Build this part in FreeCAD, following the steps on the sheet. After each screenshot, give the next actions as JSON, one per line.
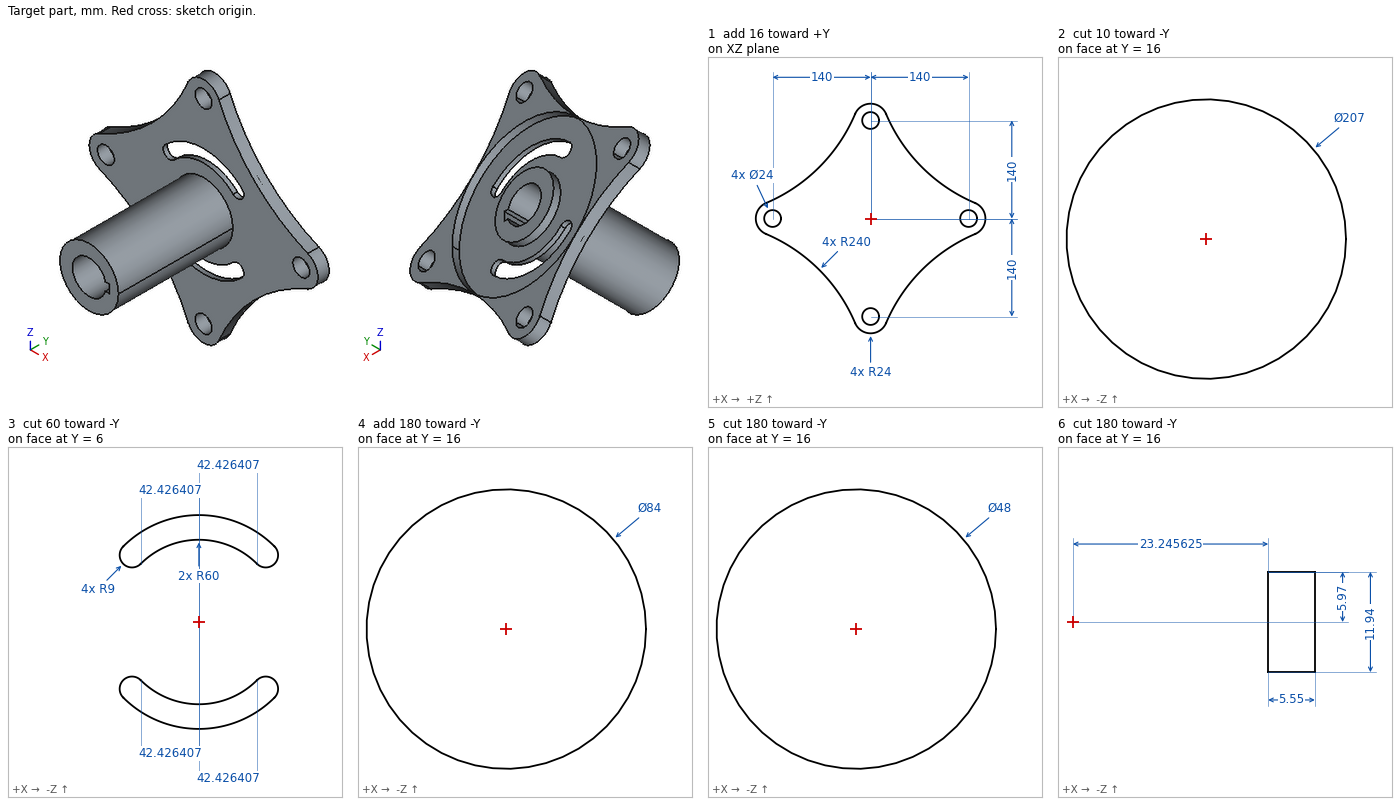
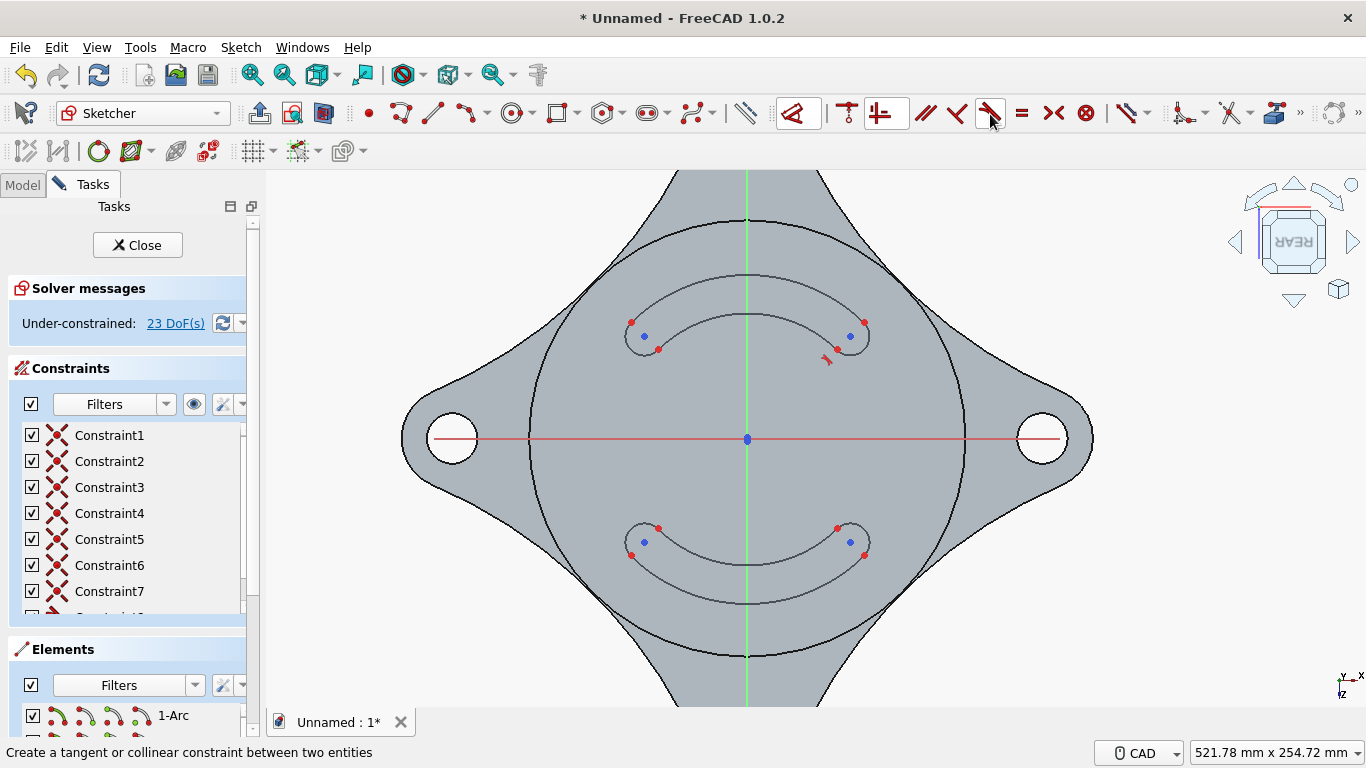
{"action": "left_click", "coordinate": [787, 320]}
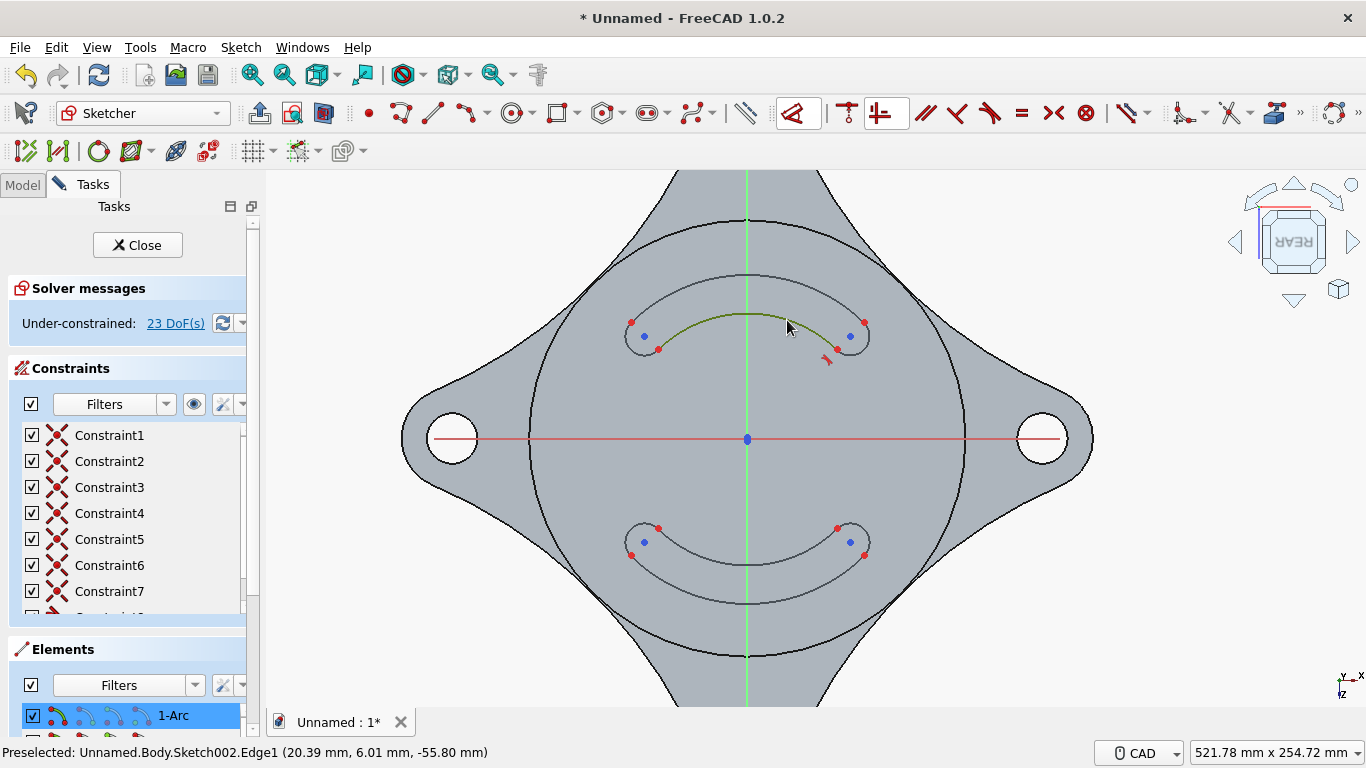
{"action": "left_click", "coordinate": [626, 339]}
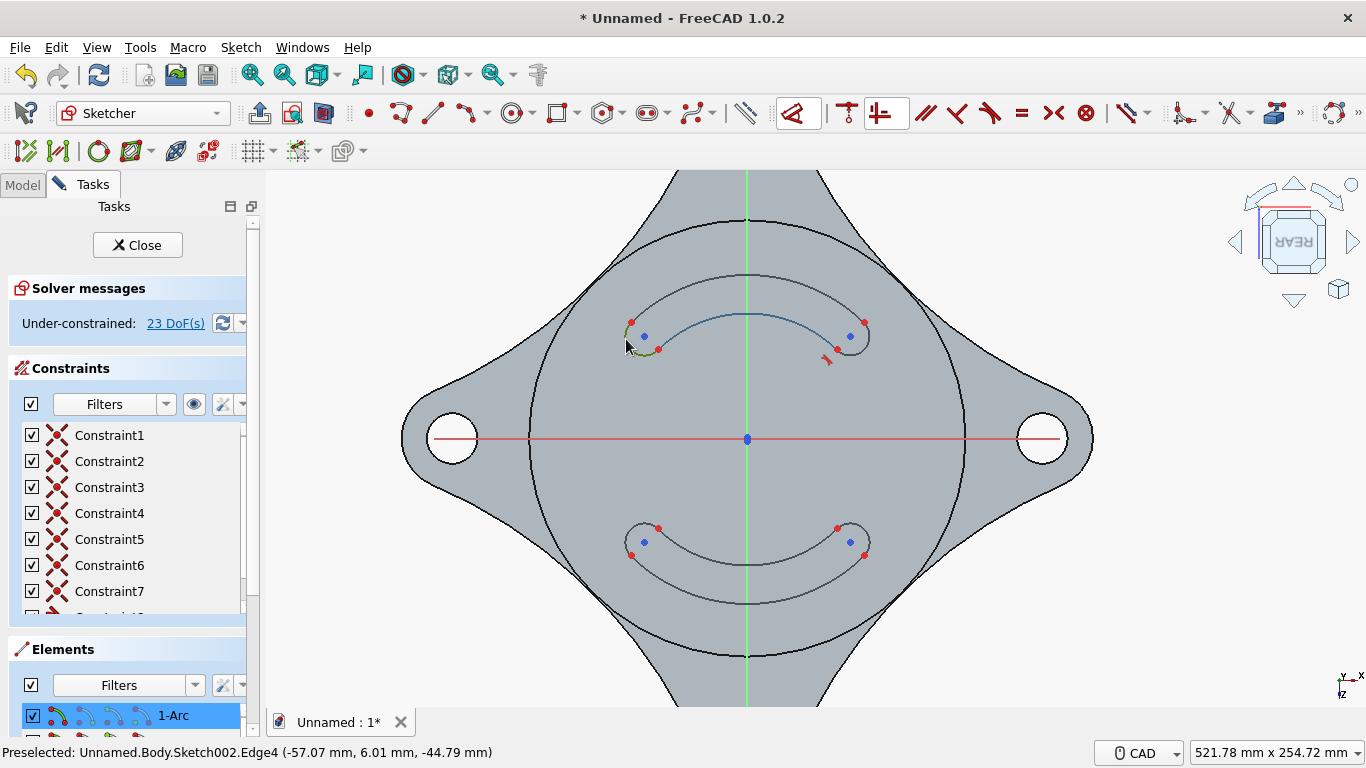
{"action": "left_click", "coordinate": [990, 114]}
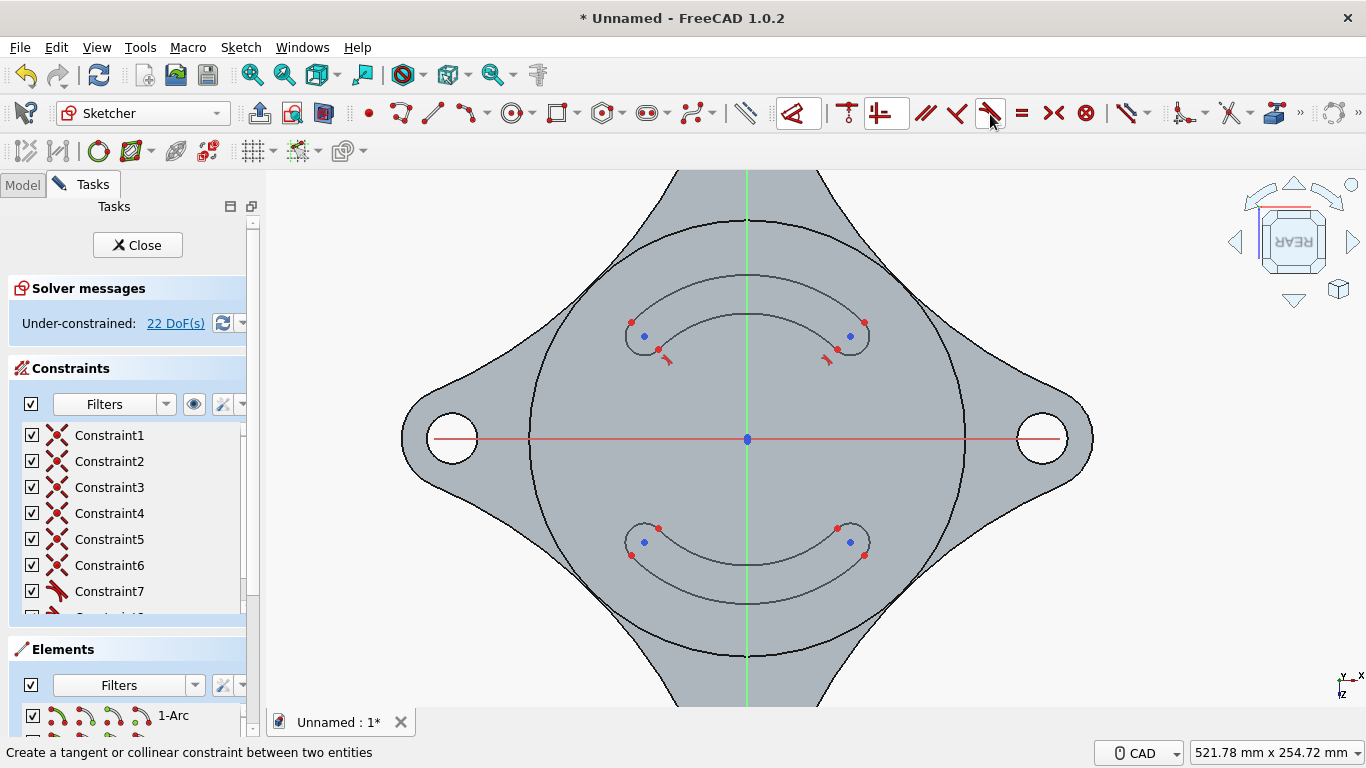
{"action": "left_click", "coordinate": [853, 355]}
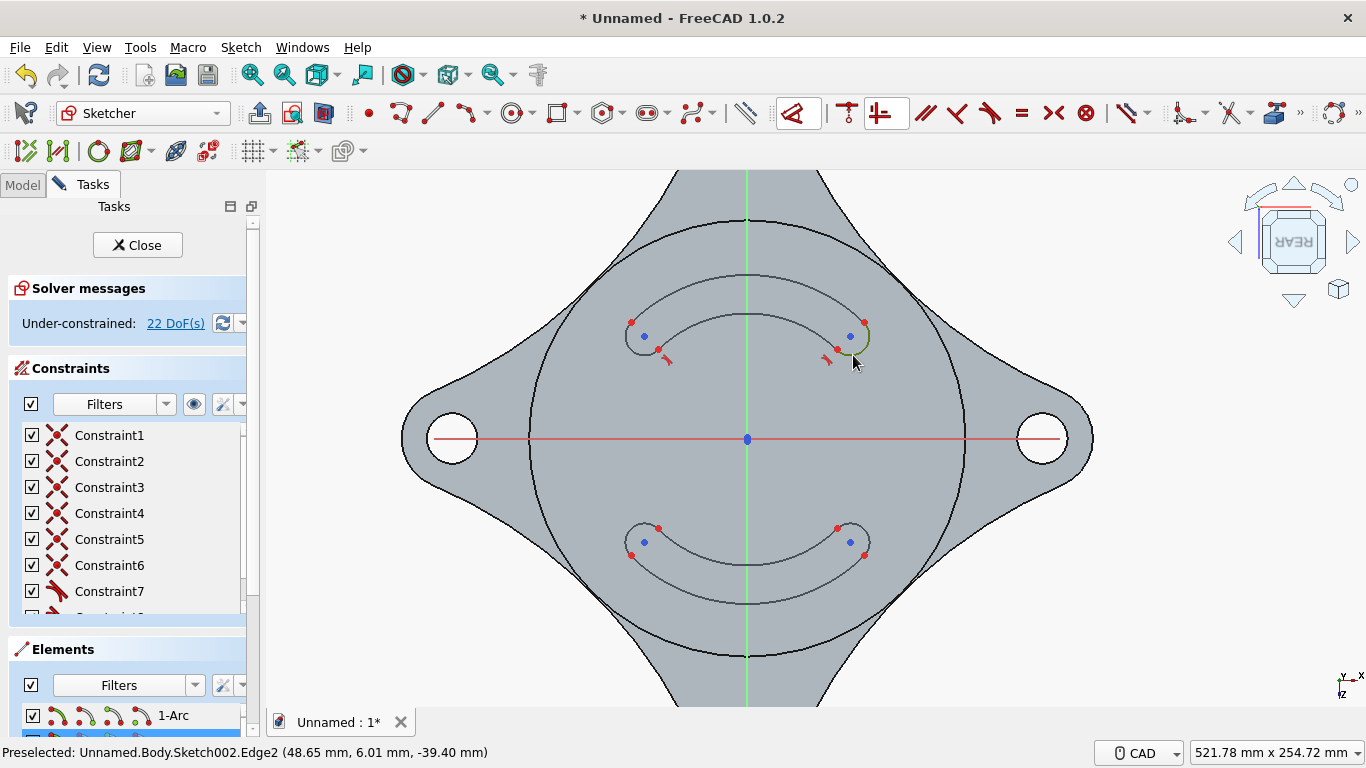
{"action": "left_click", "coordinate": [798, 283]}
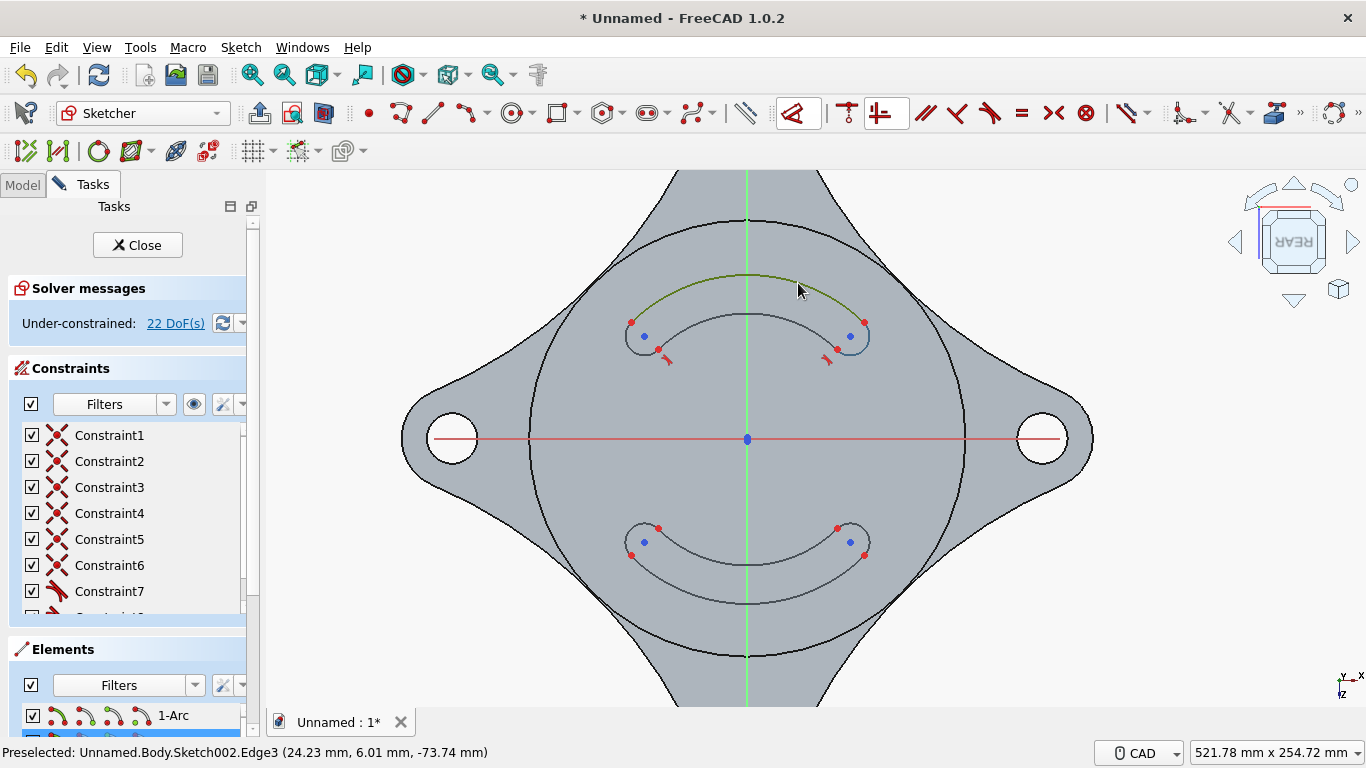
{"action": "left_click", "coordinate": [990, 114]}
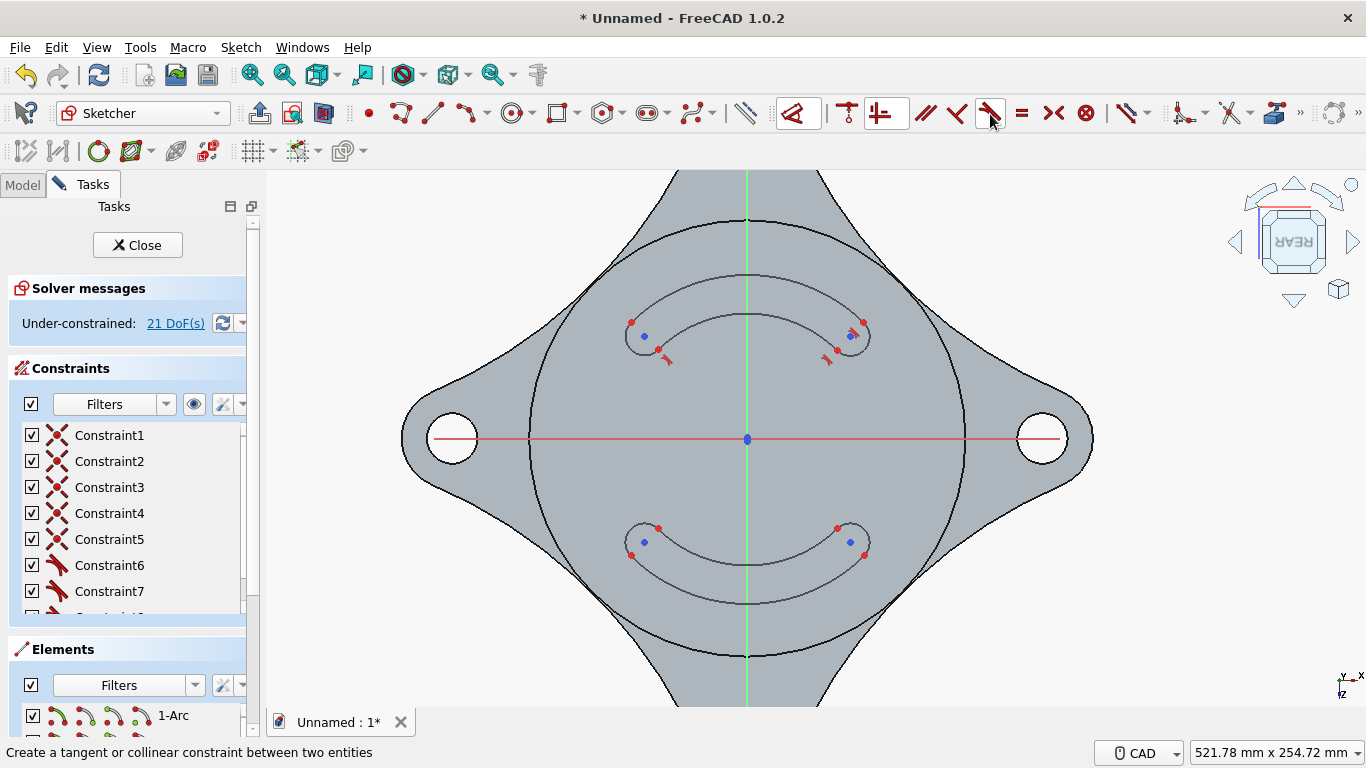
{"action": "left_click", "coordinate": [798, 283]}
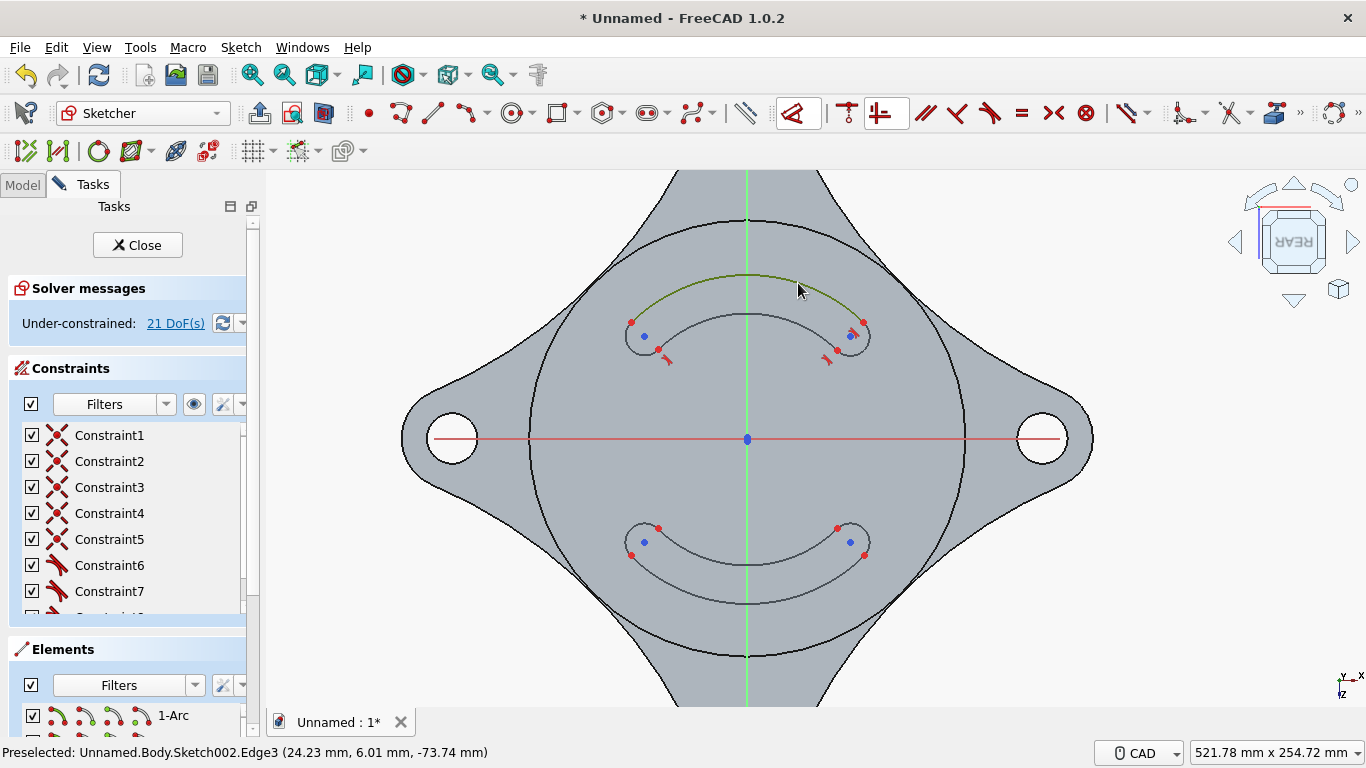
{"action": "left_click", "coordinate": [626, 339]}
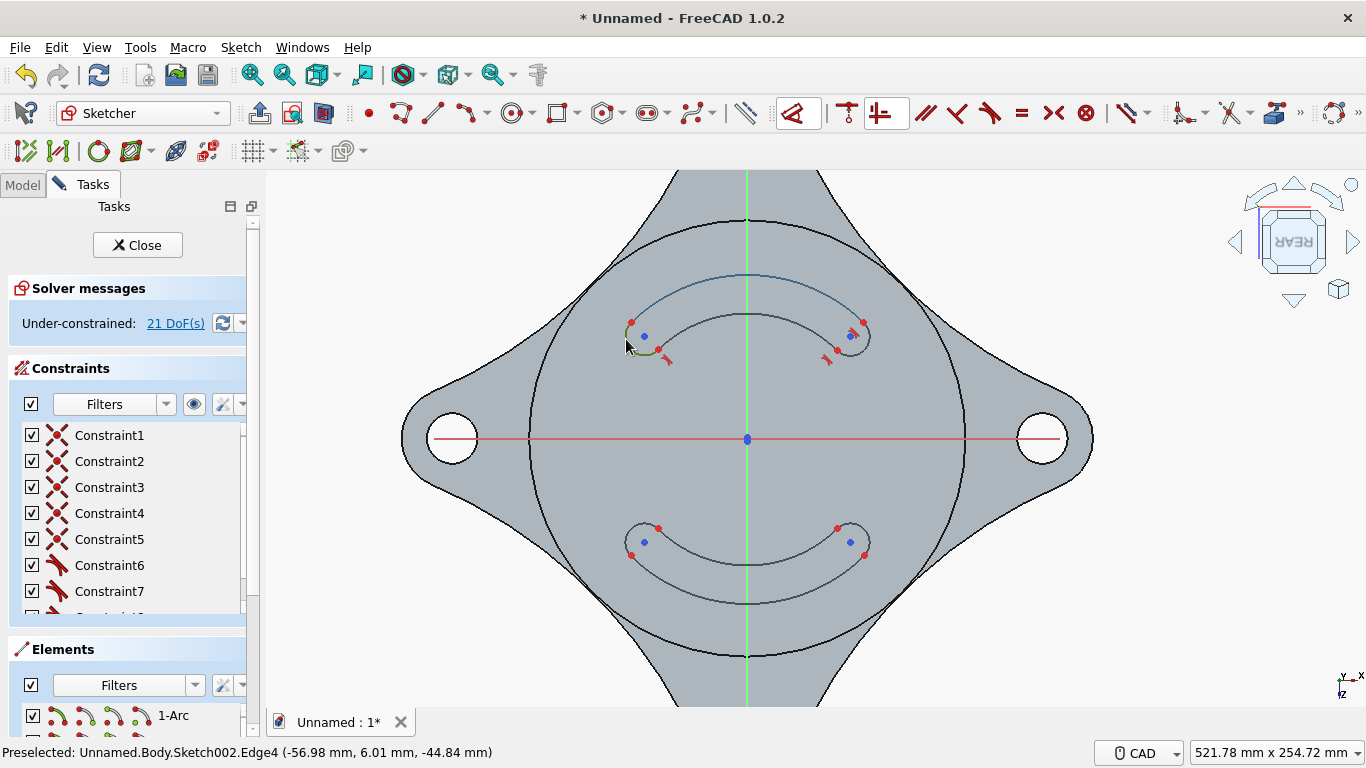
{"action": "left_click", "coordinate": [990, 114]}